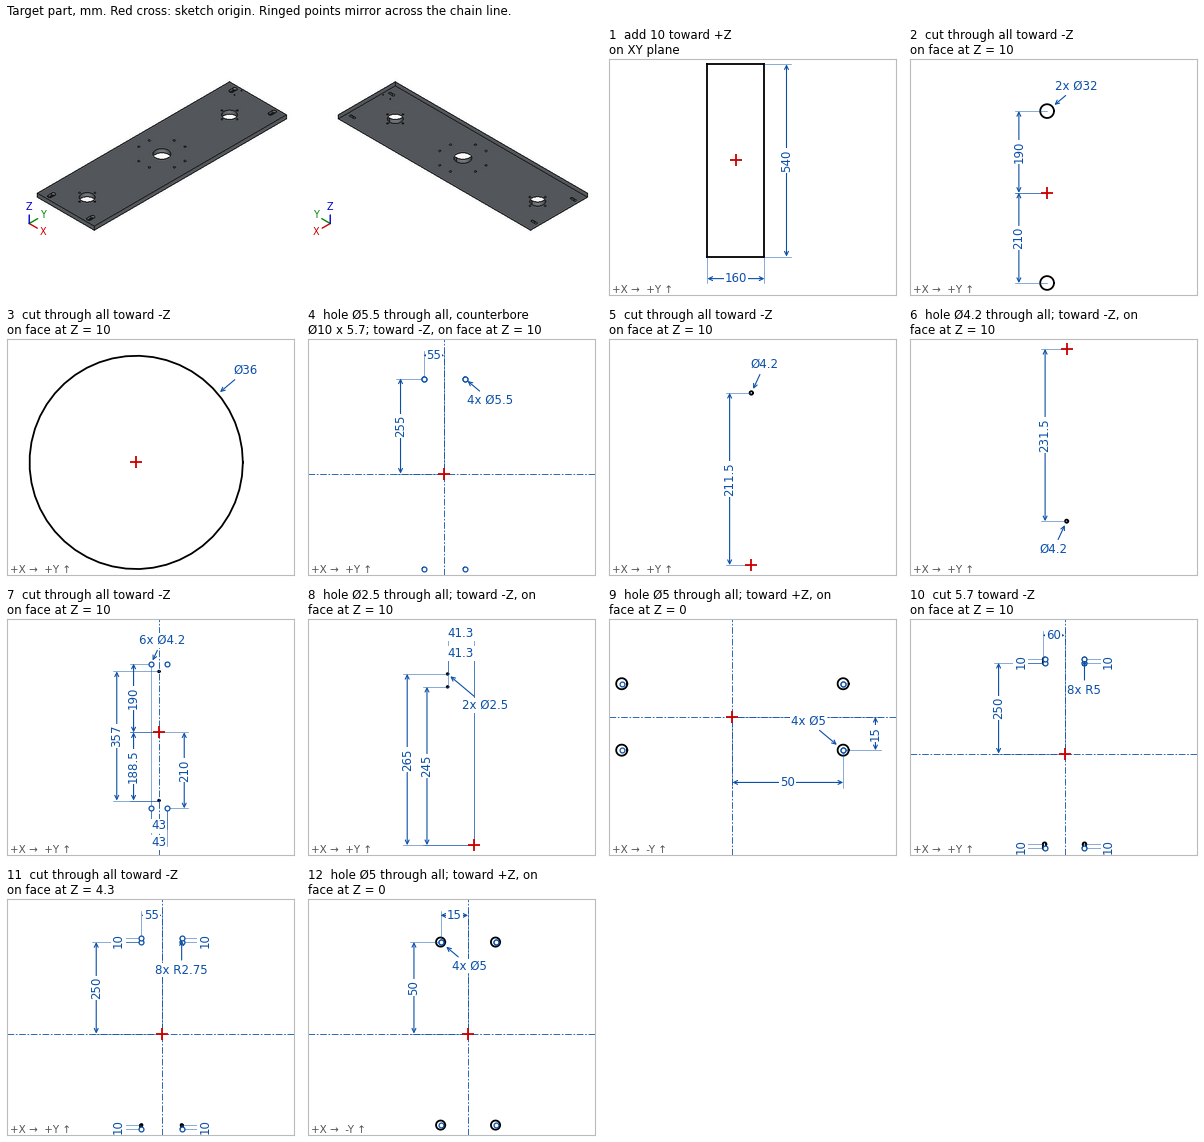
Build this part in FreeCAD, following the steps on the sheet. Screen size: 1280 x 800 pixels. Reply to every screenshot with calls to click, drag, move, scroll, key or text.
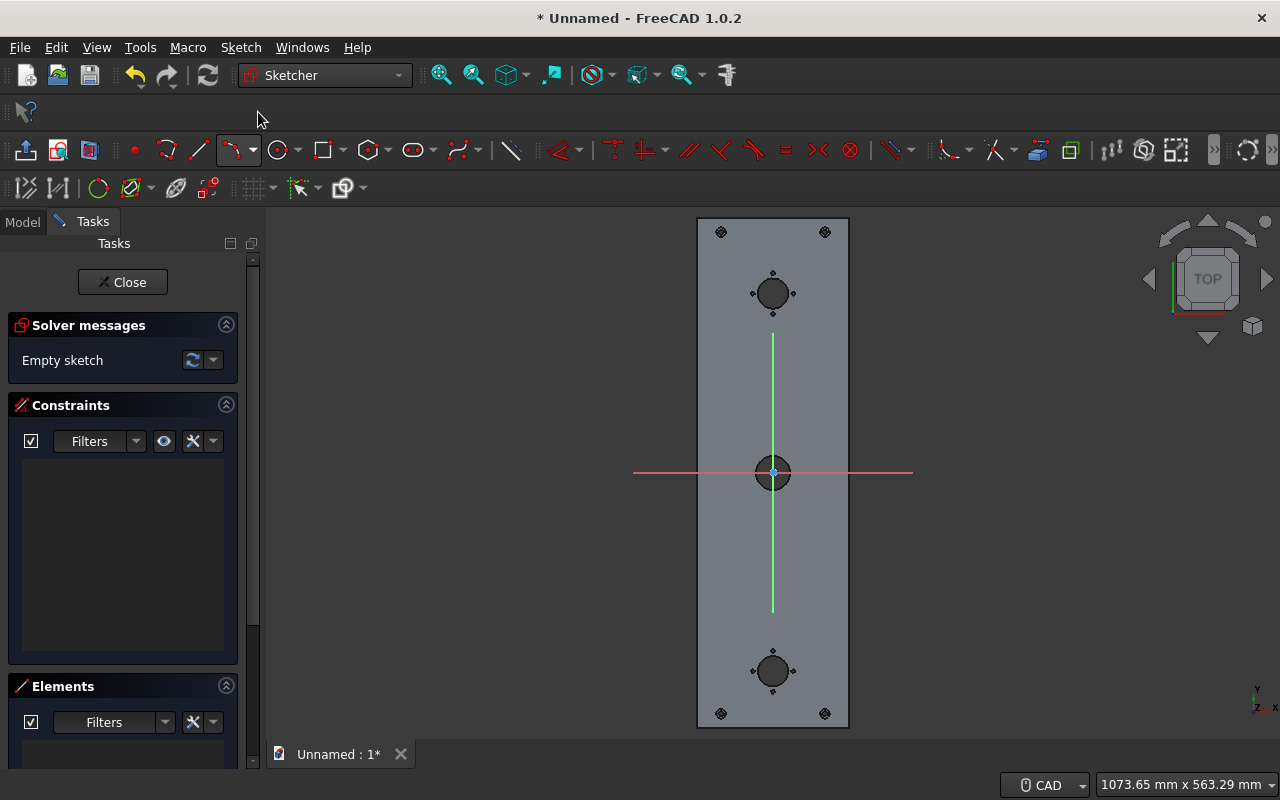
scroll(704, 473, down, 5)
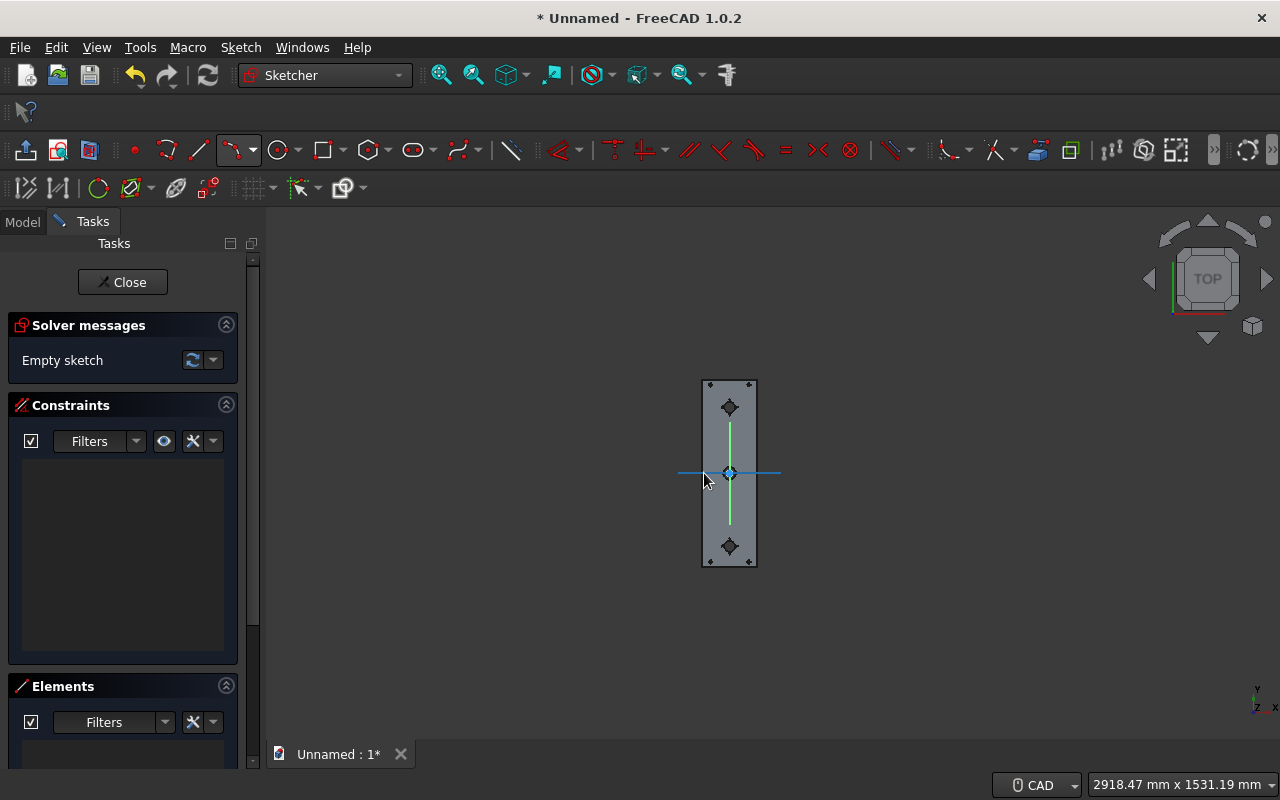
scroll(716, 380, up, 15)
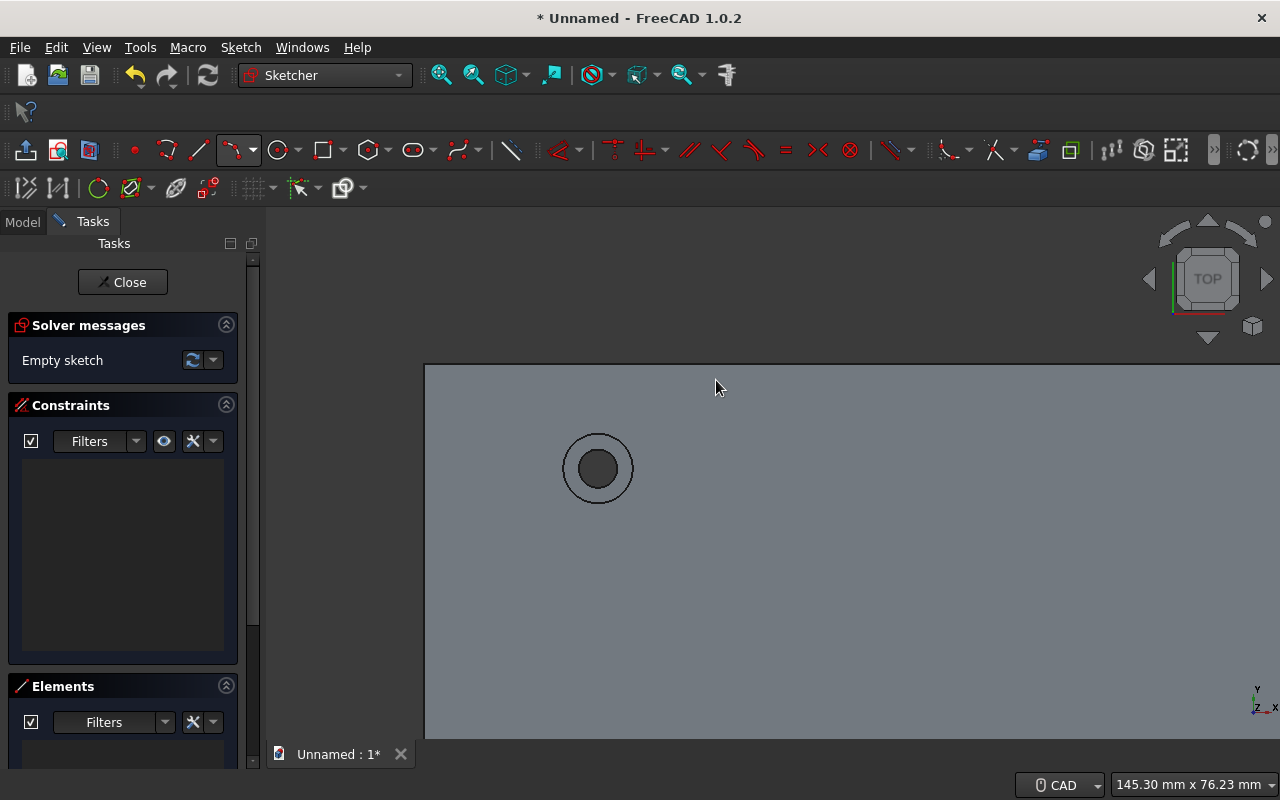
scroll(685, 465, up, 4)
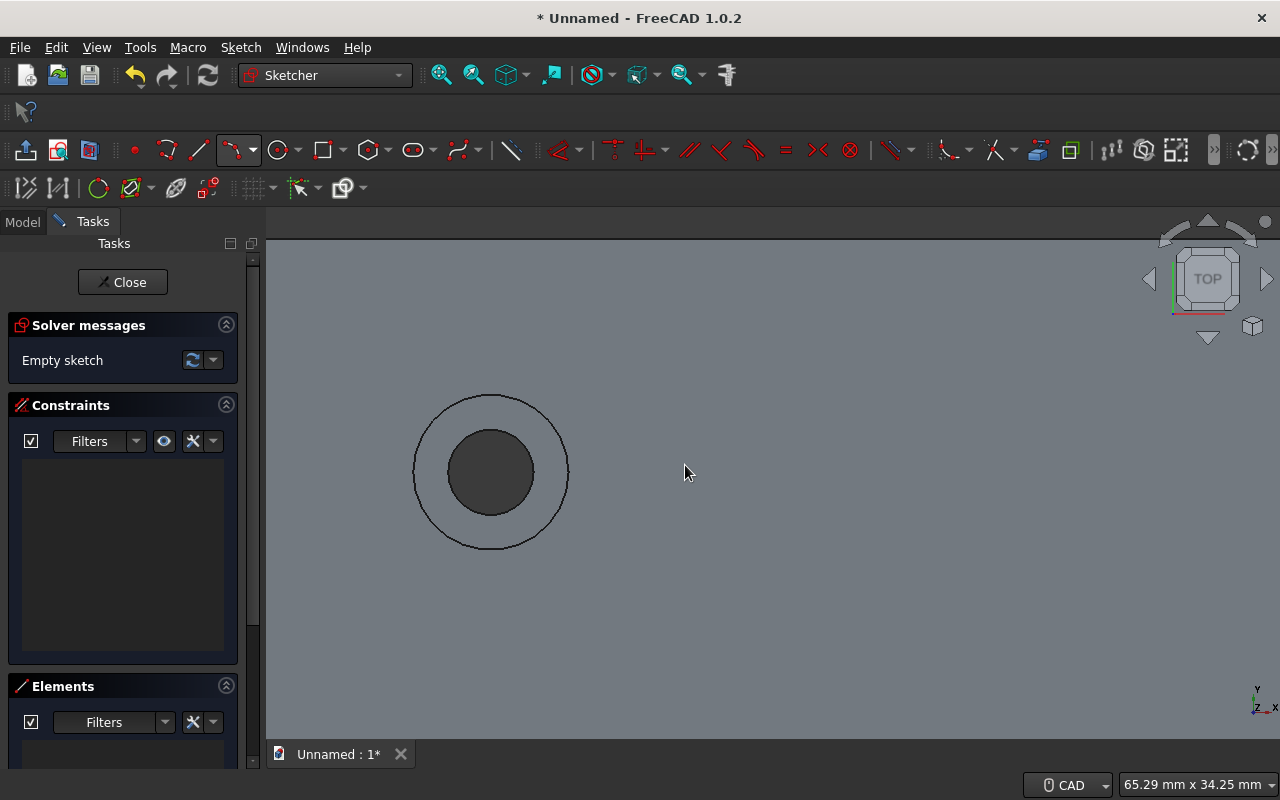
key(g)
key(c)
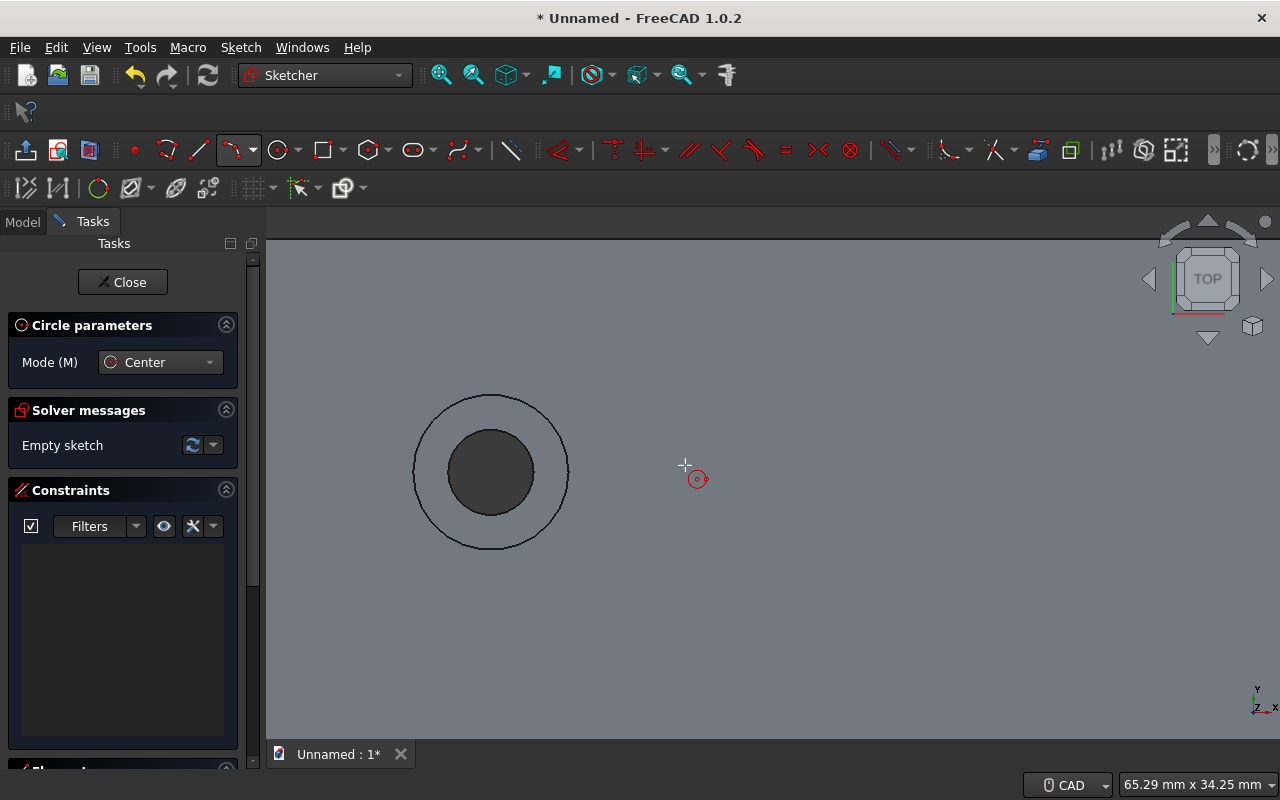
click(704, 317)
move(717, 303)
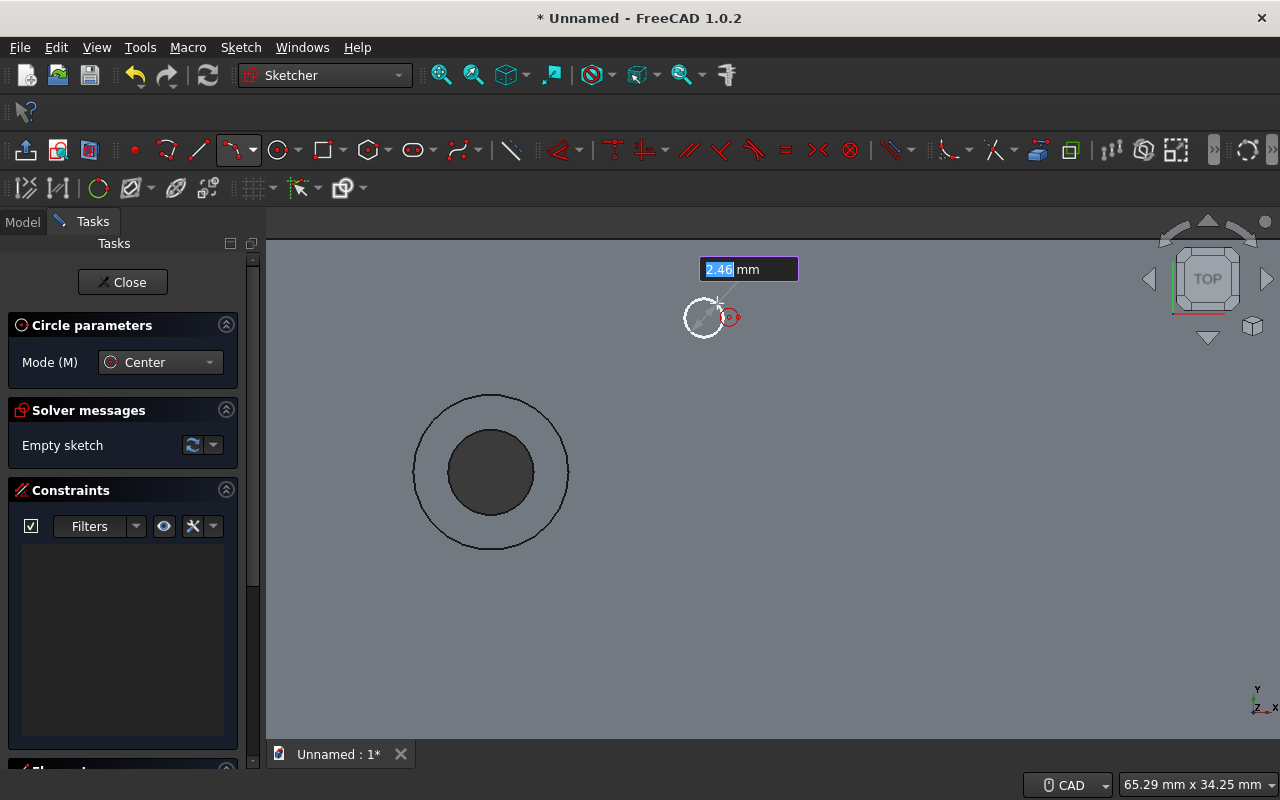
text(2.5)
key(Return)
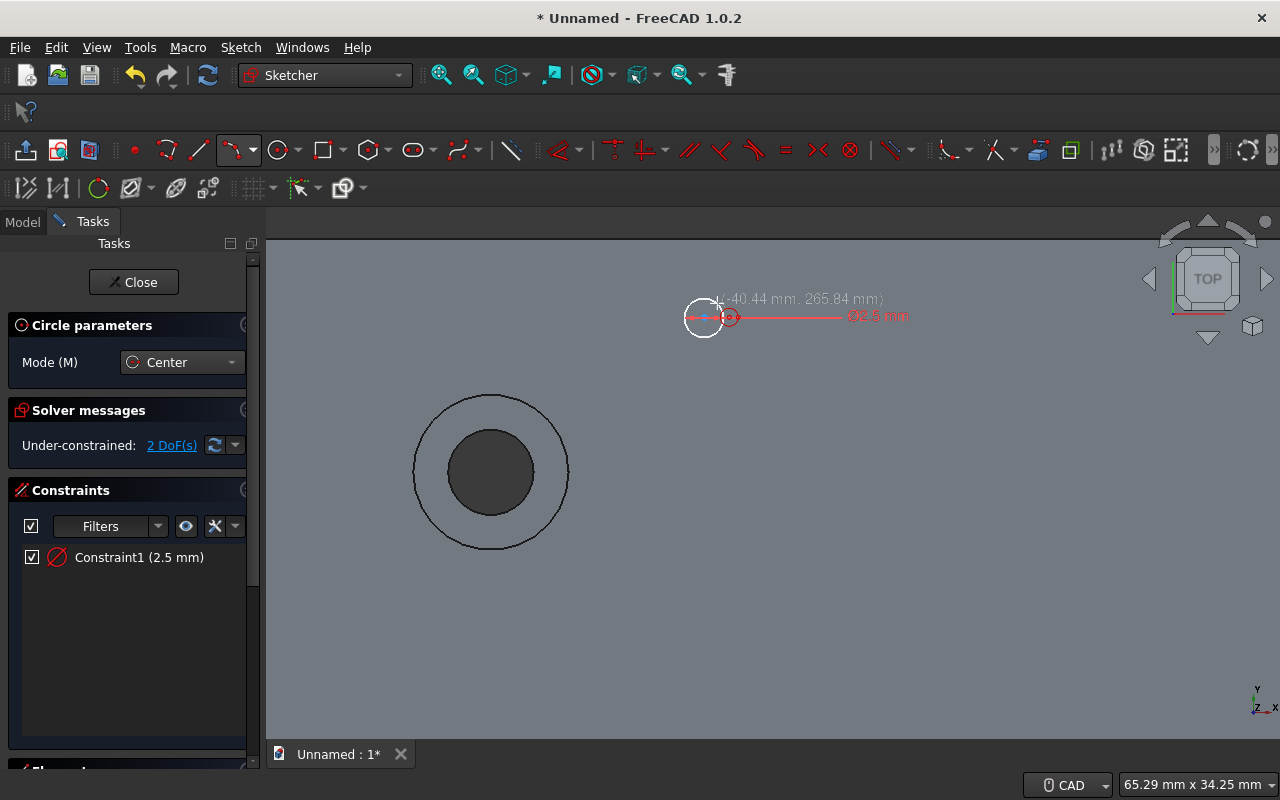
click(704, 628)
move(717, 614)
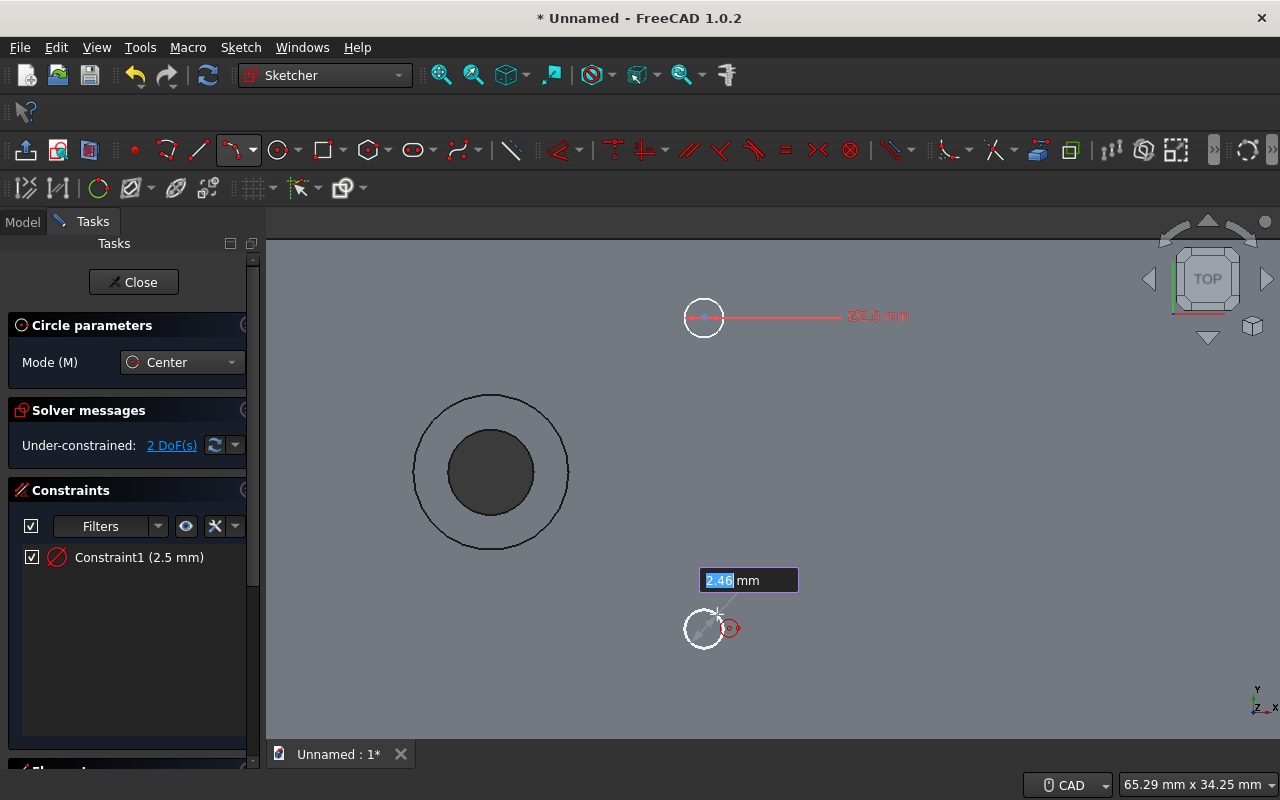
text(2.5)
key(Return)
key(Escape)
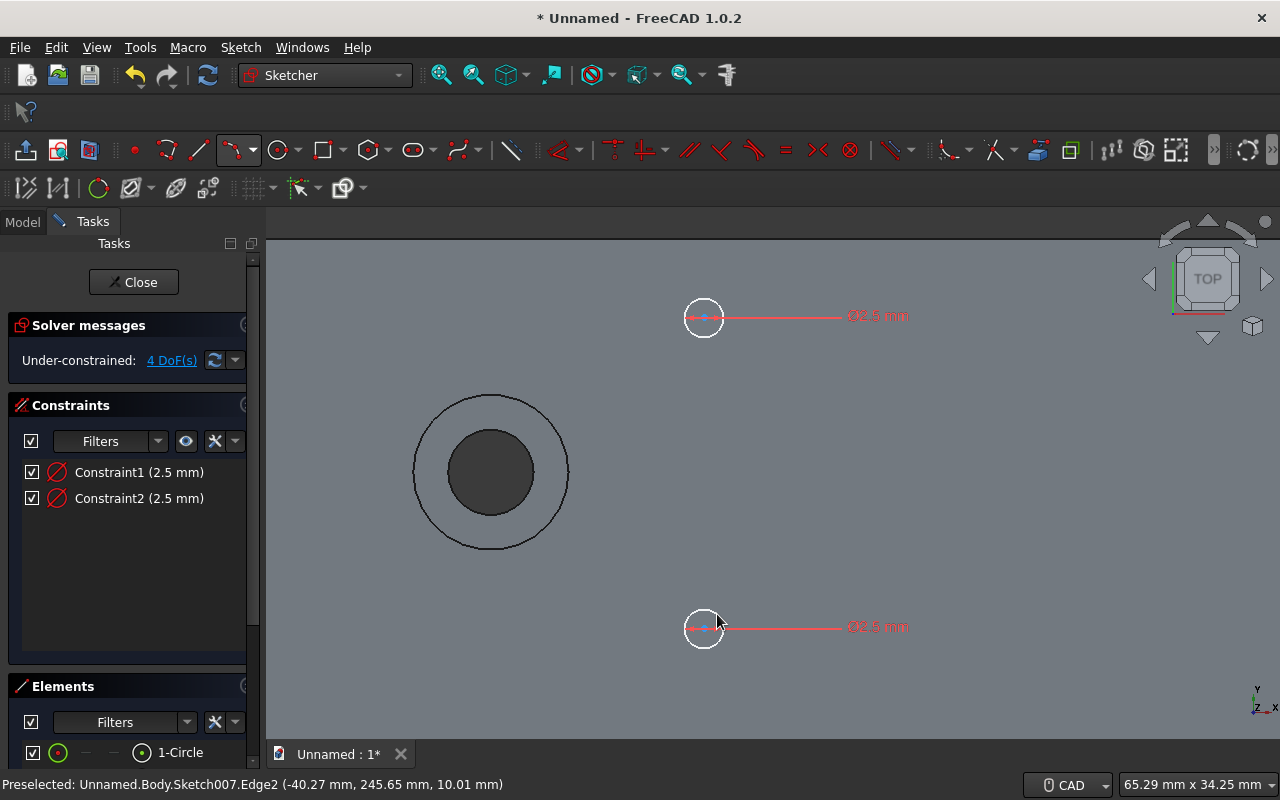
key(d)